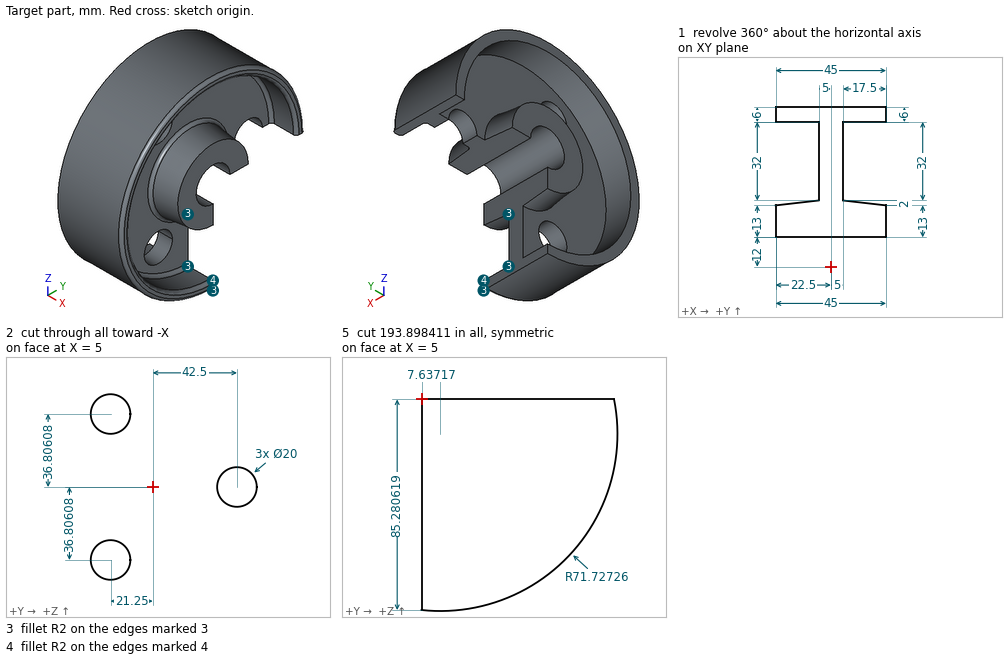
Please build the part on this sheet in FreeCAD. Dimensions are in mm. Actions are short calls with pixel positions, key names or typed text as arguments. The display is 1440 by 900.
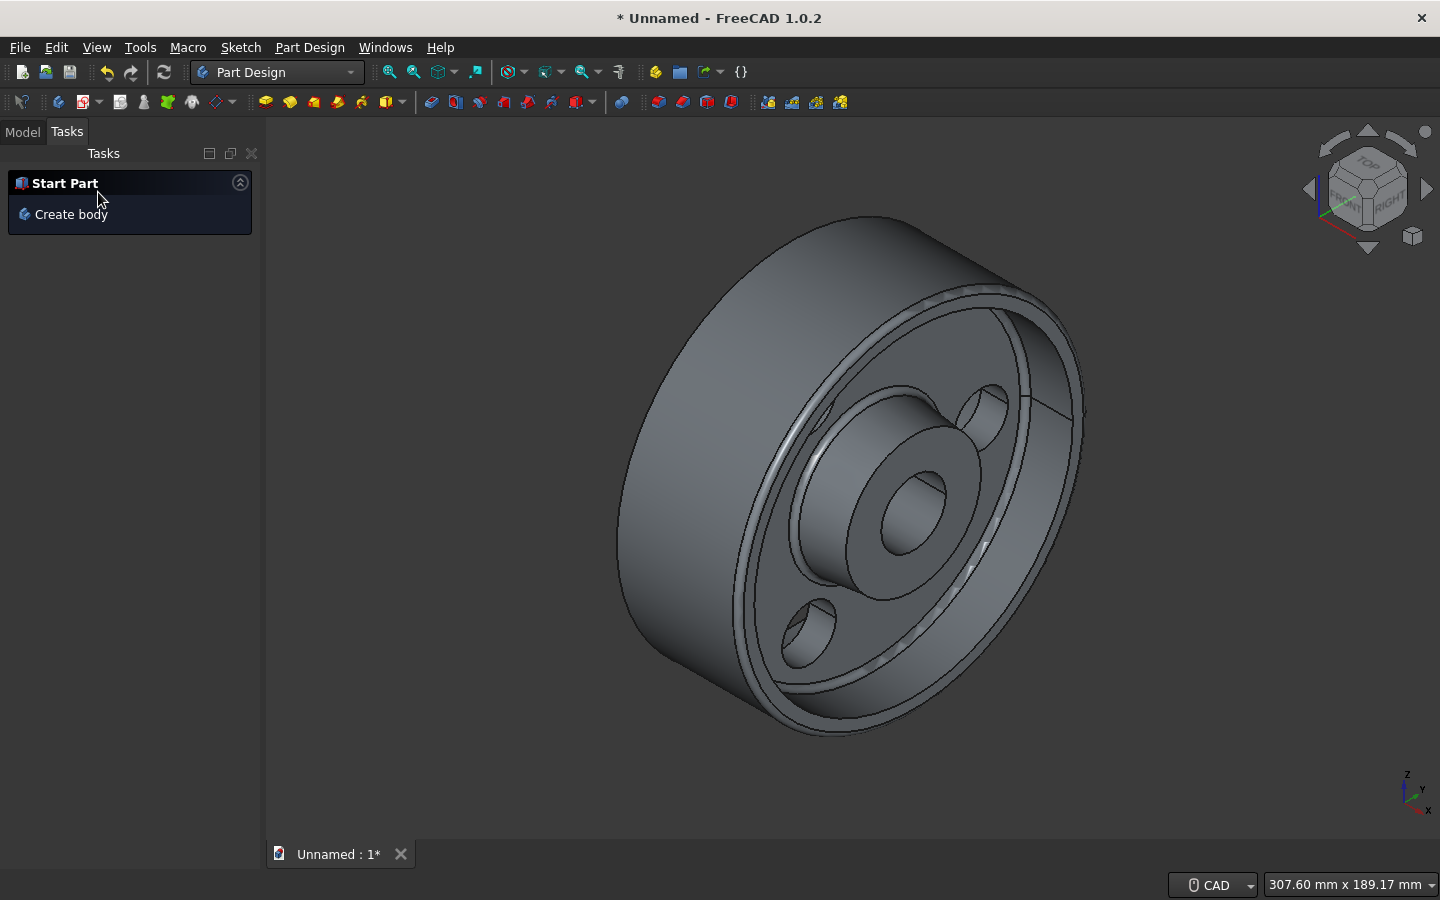
click(864, 715)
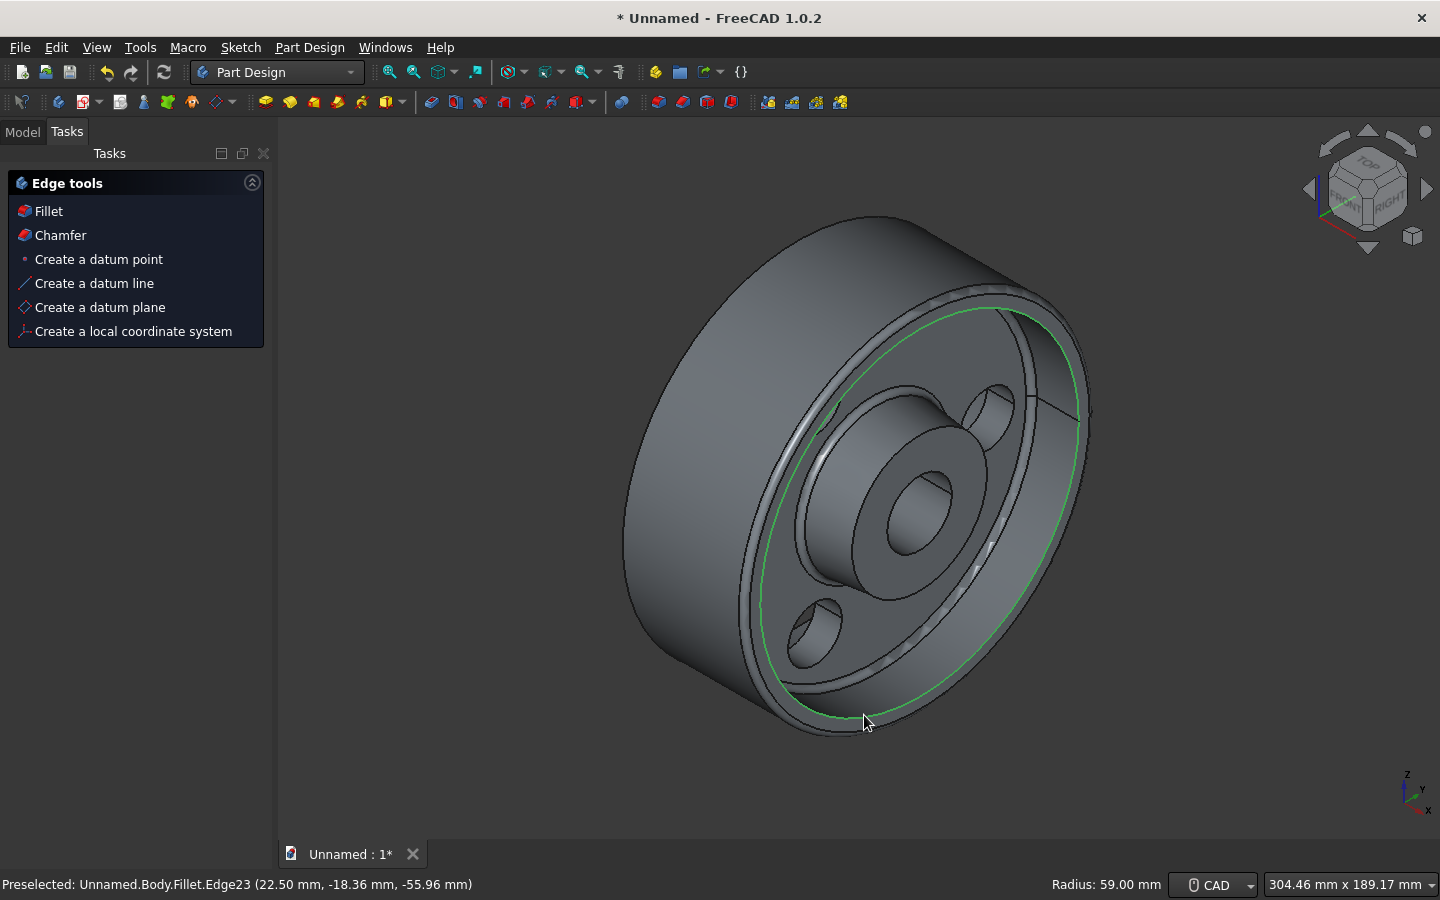
click(660, 102)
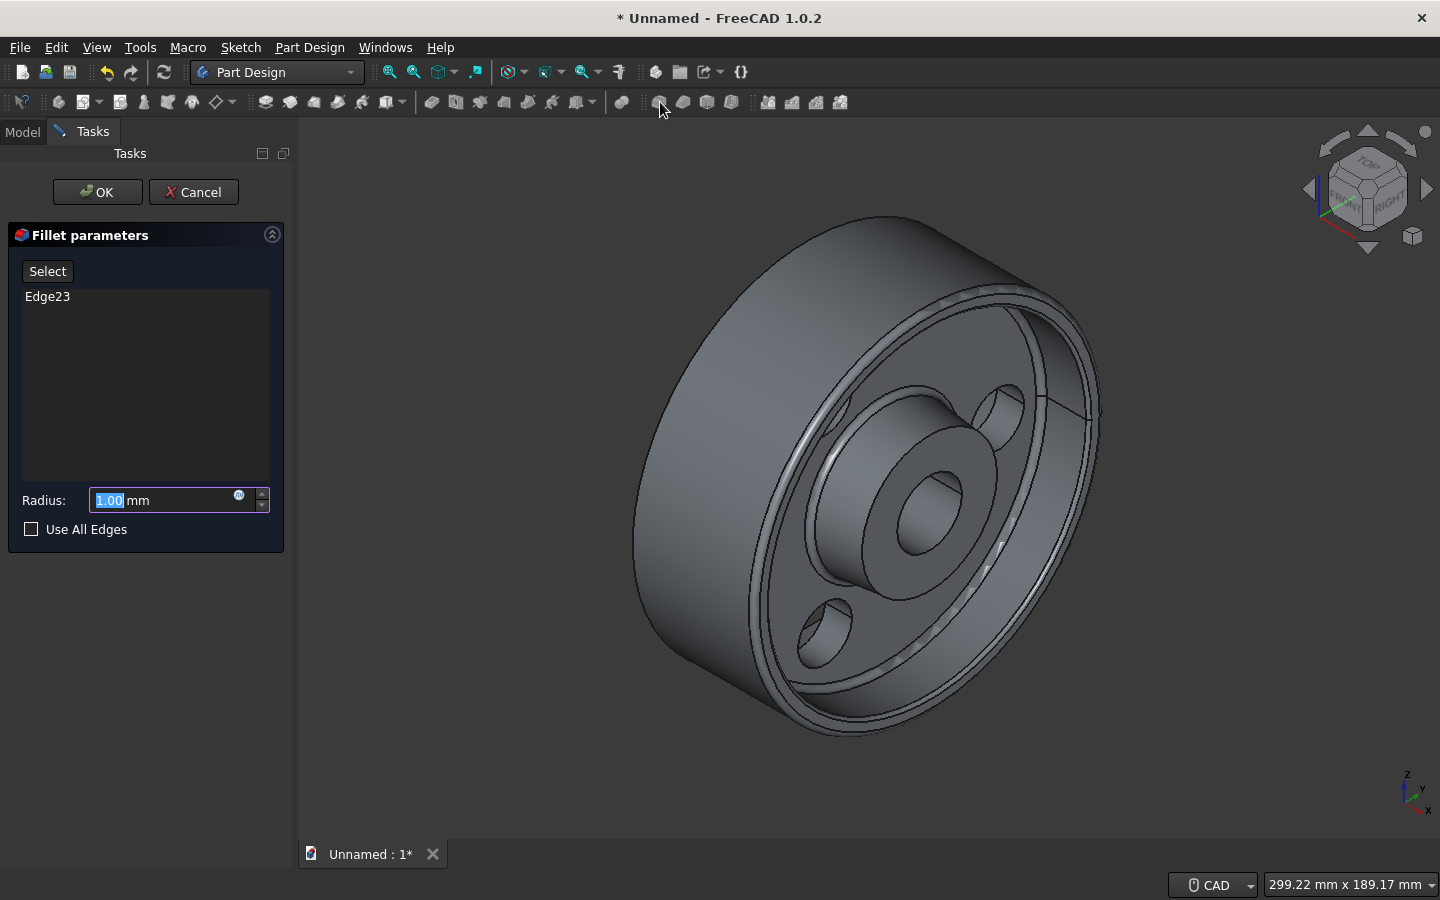
text(2)
key(Tab)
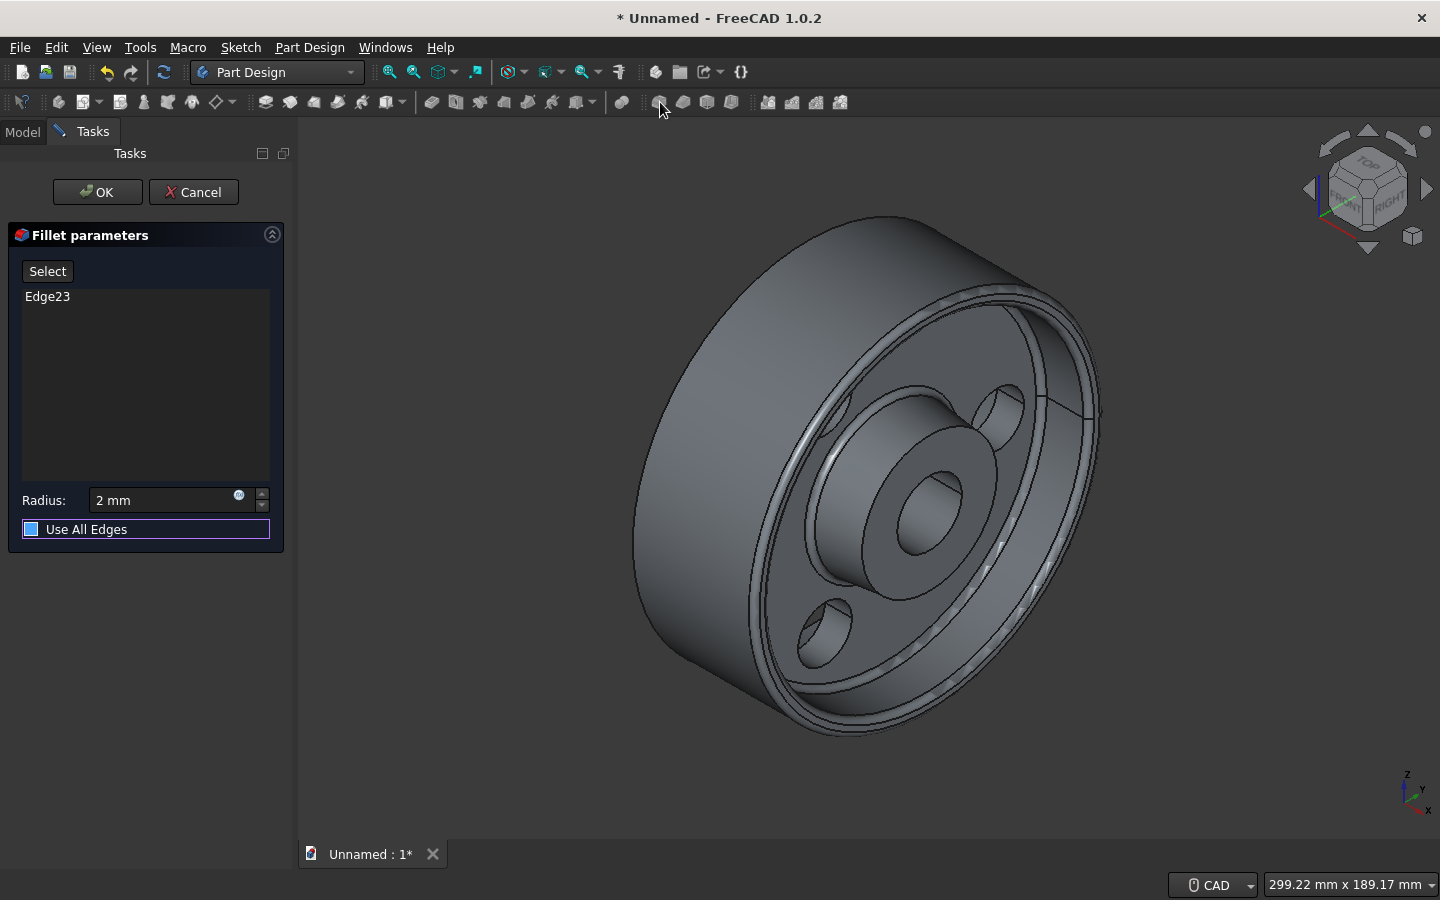
click(98, 192)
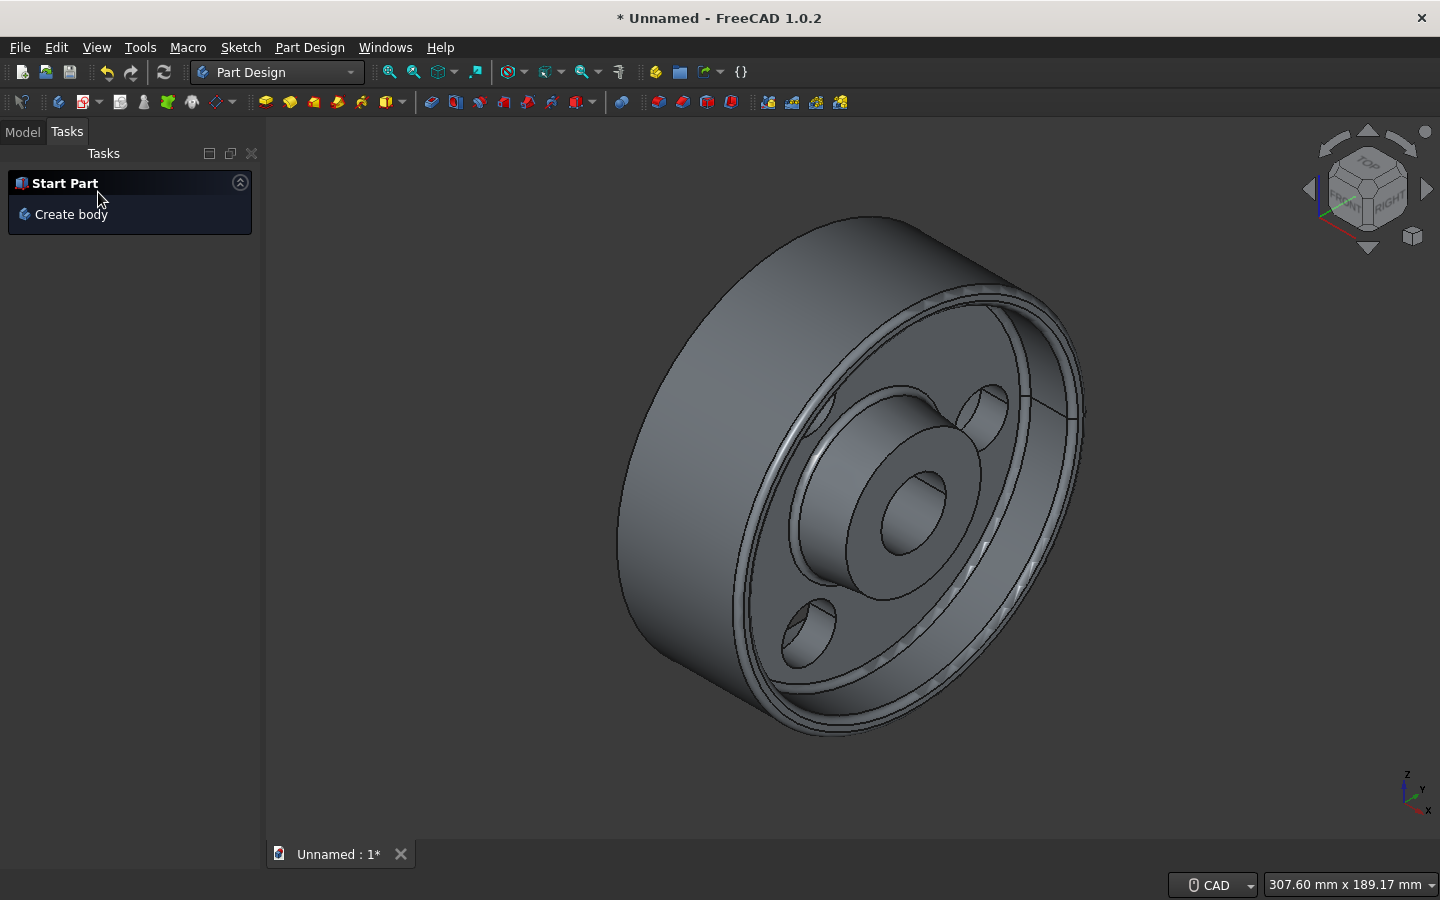
click(954, 333)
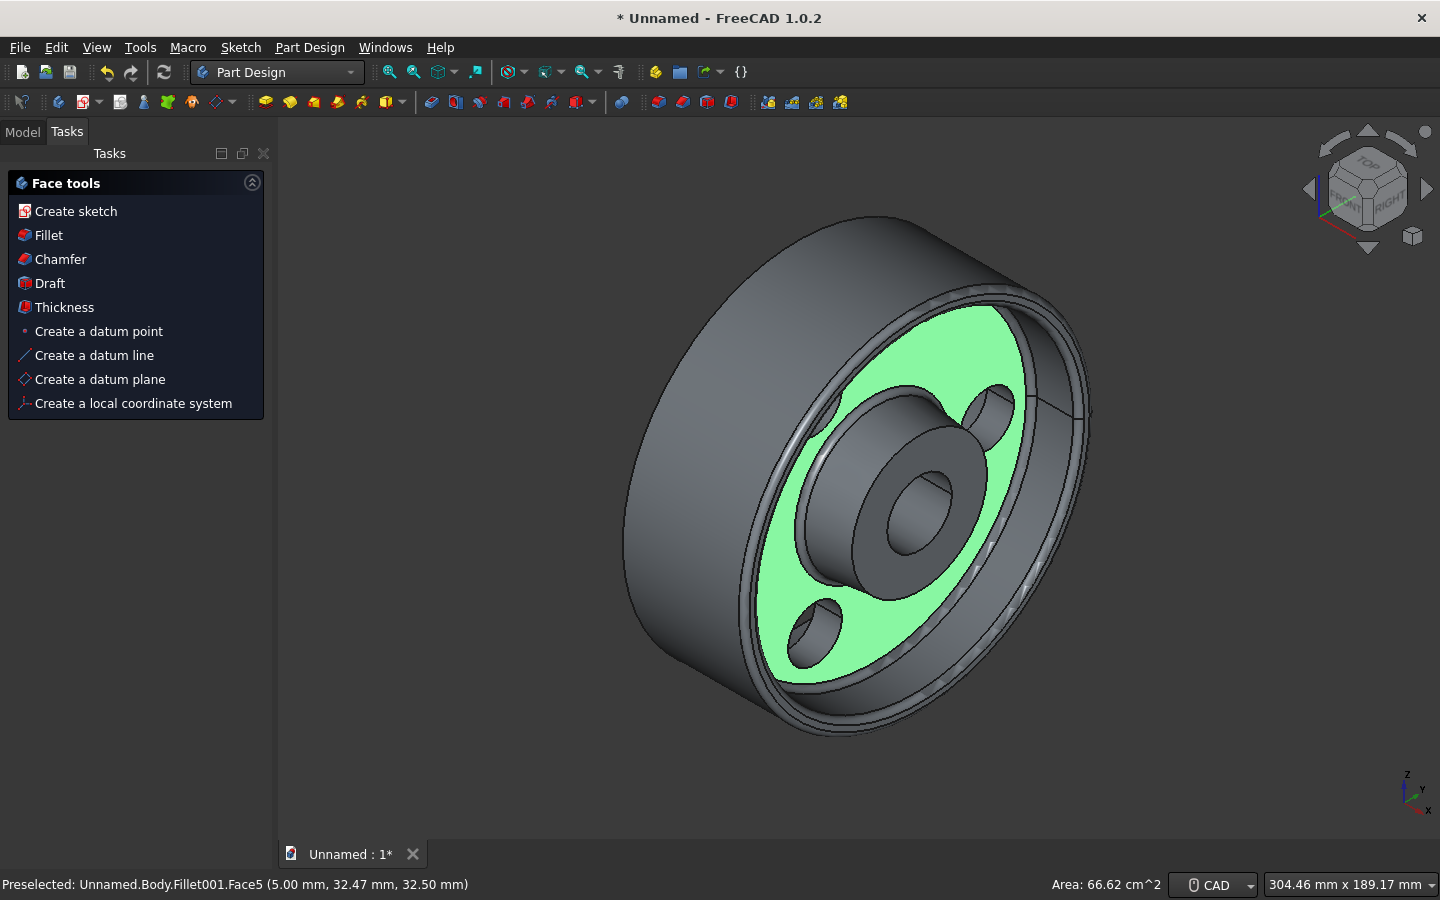
click(84, 102)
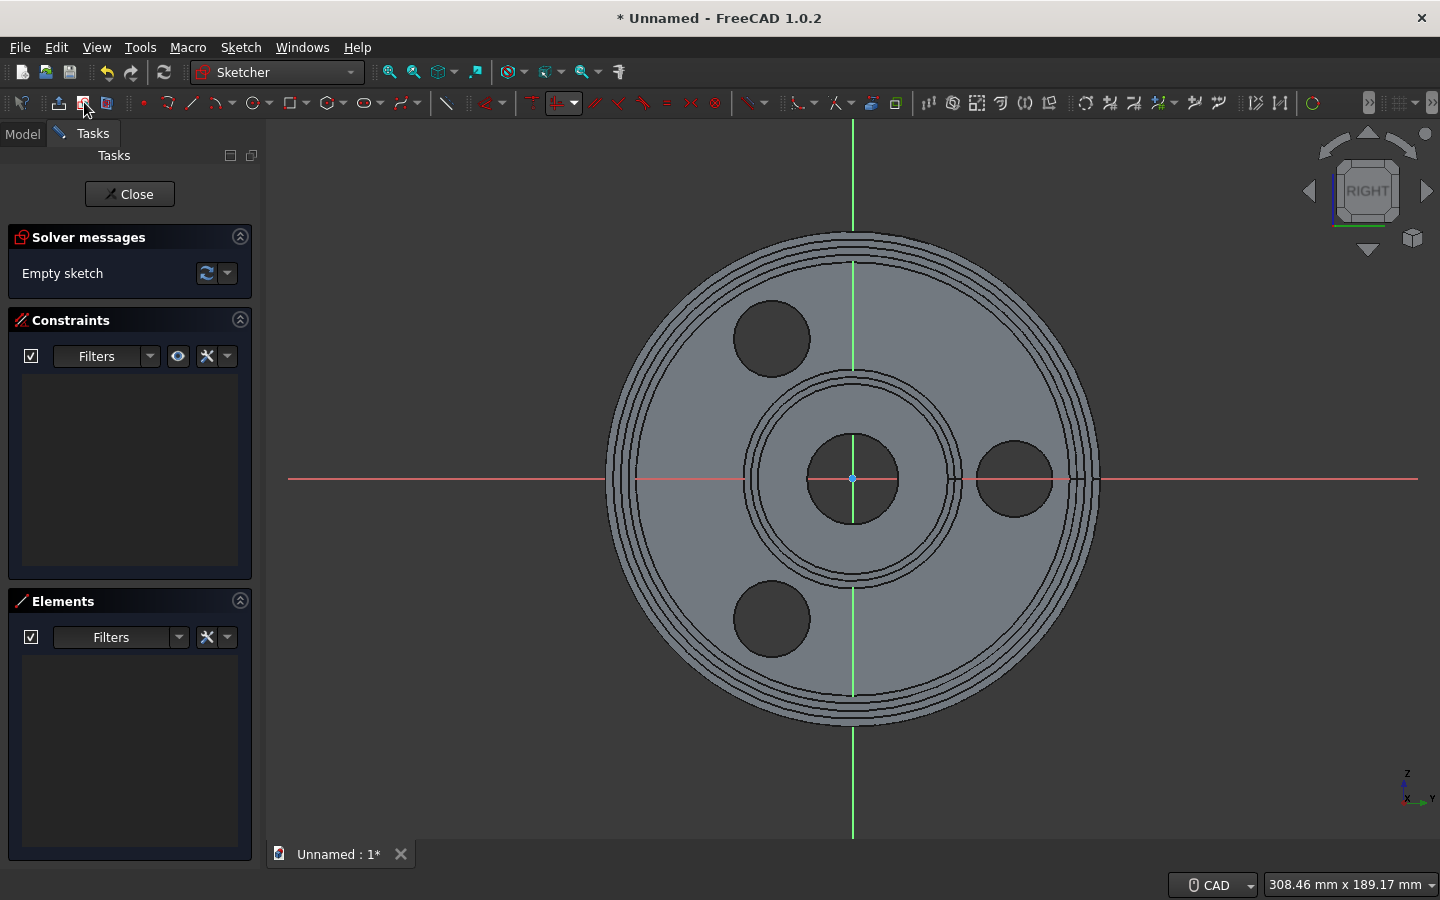
click(108, 104)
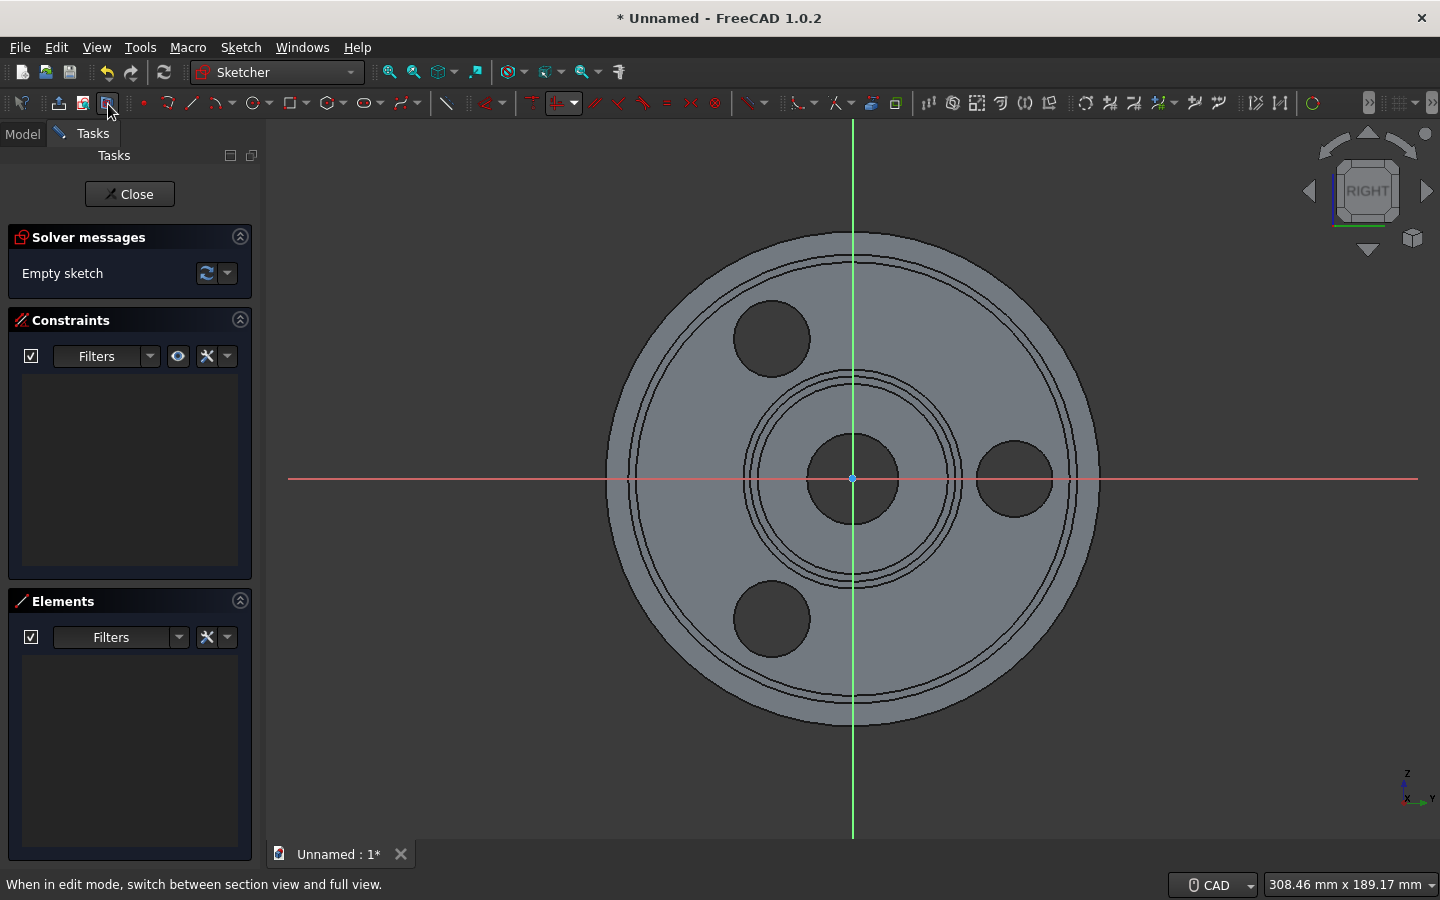
scroll(294, 147, down, 1)